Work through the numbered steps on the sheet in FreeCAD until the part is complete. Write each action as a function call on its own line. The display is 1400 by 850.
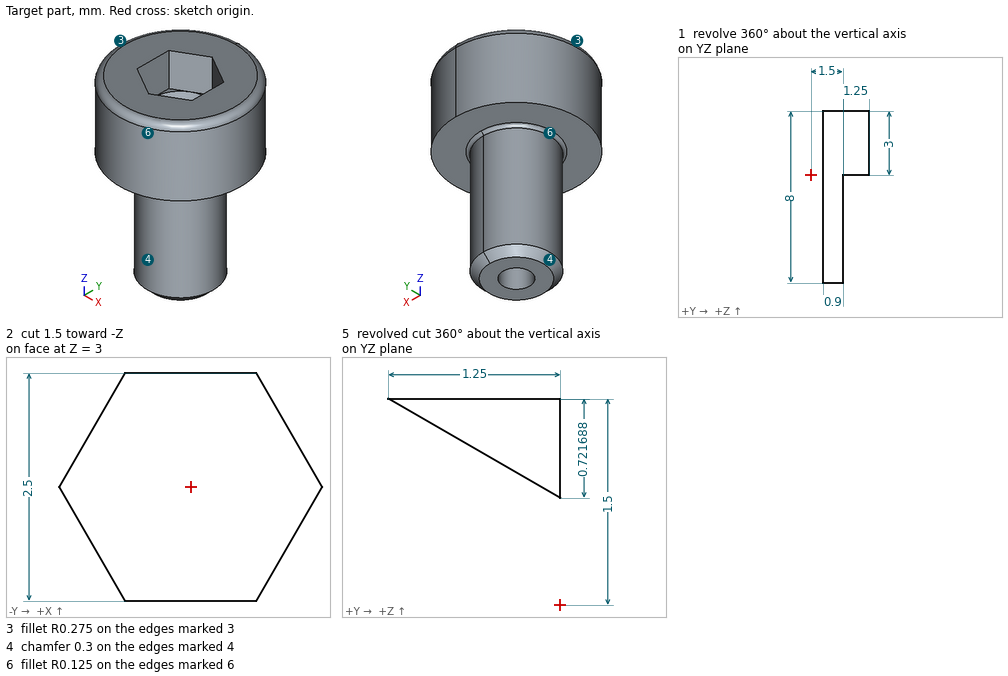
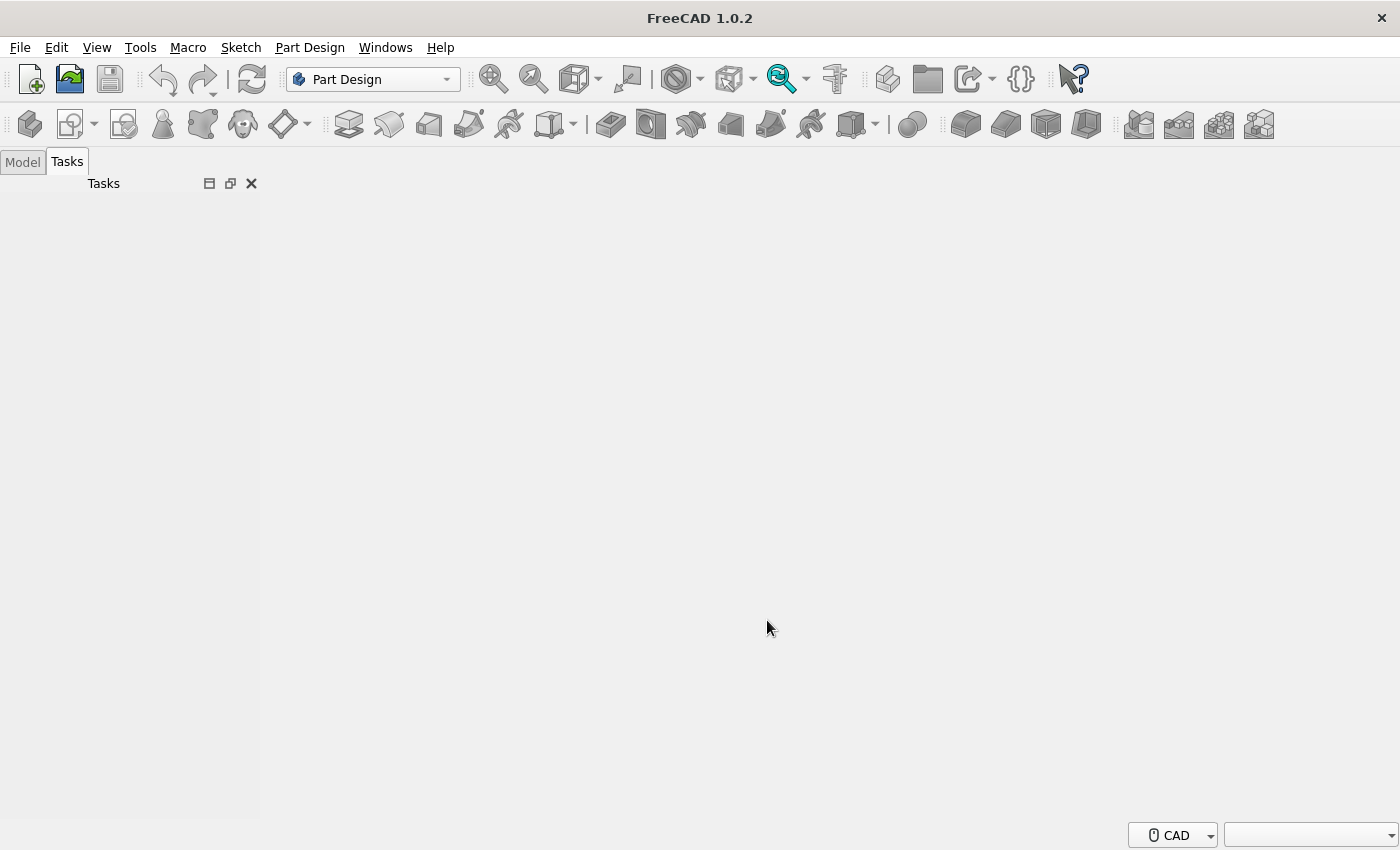
click(30, 80)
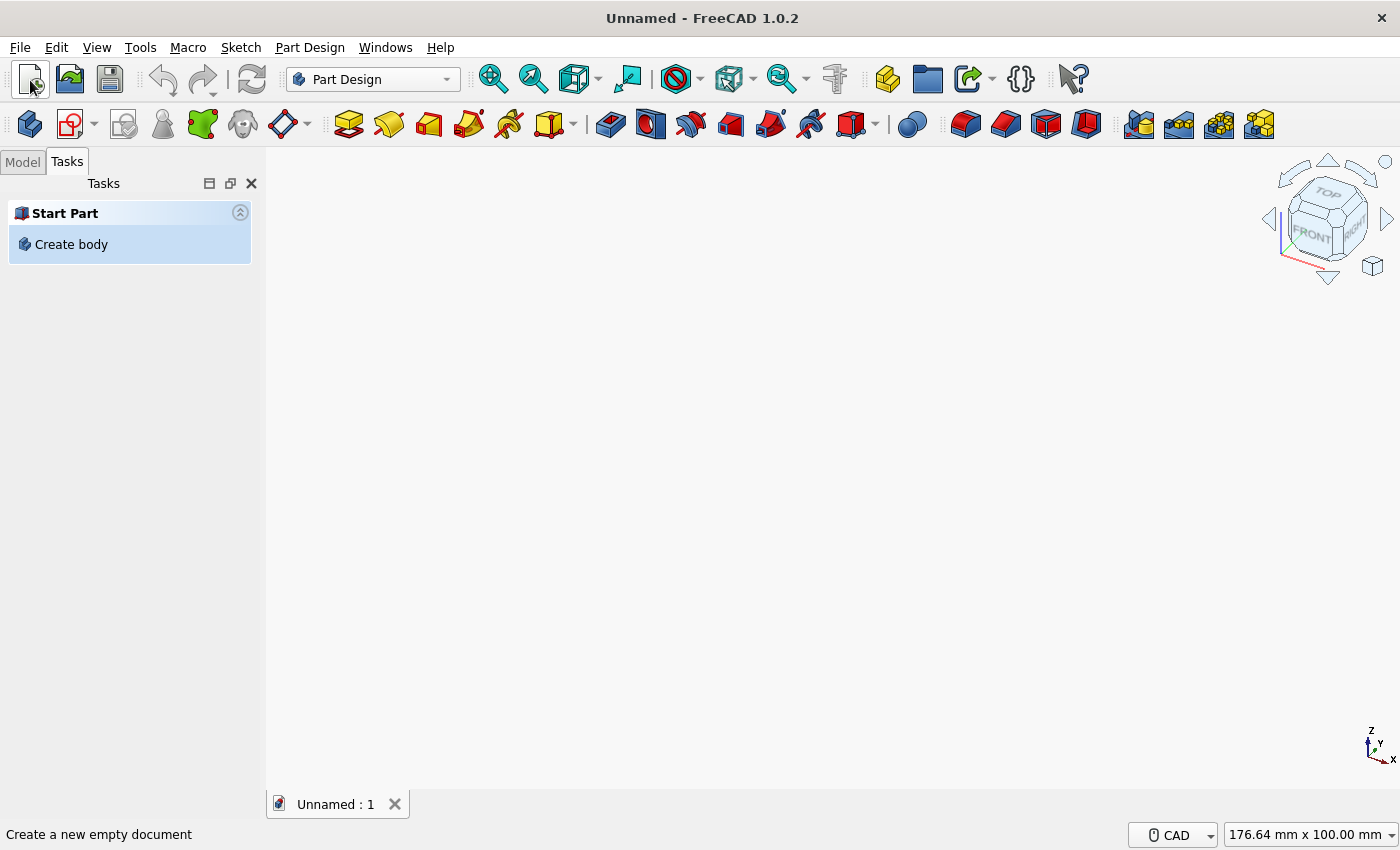
click(70, 124)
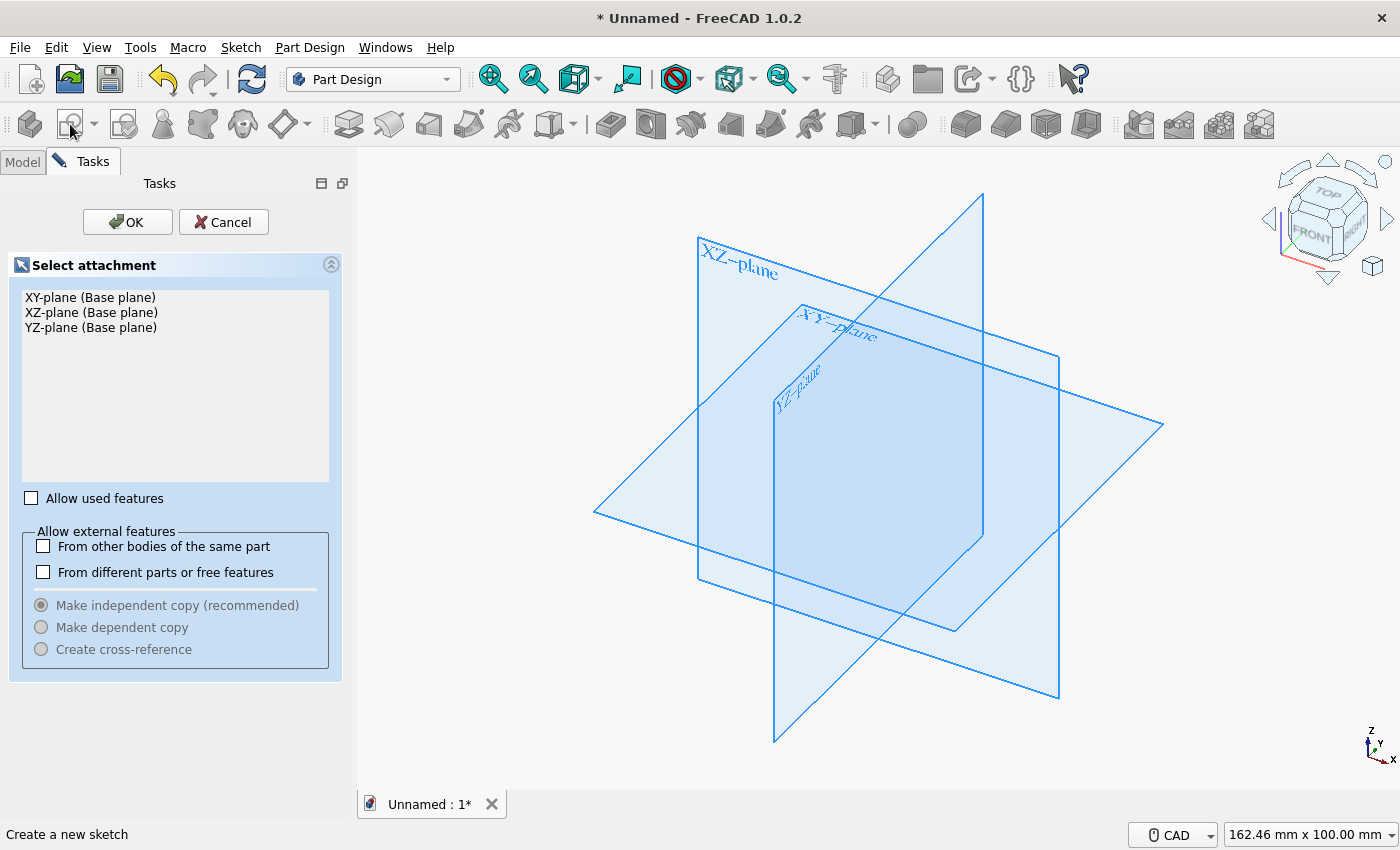
click(82, 328)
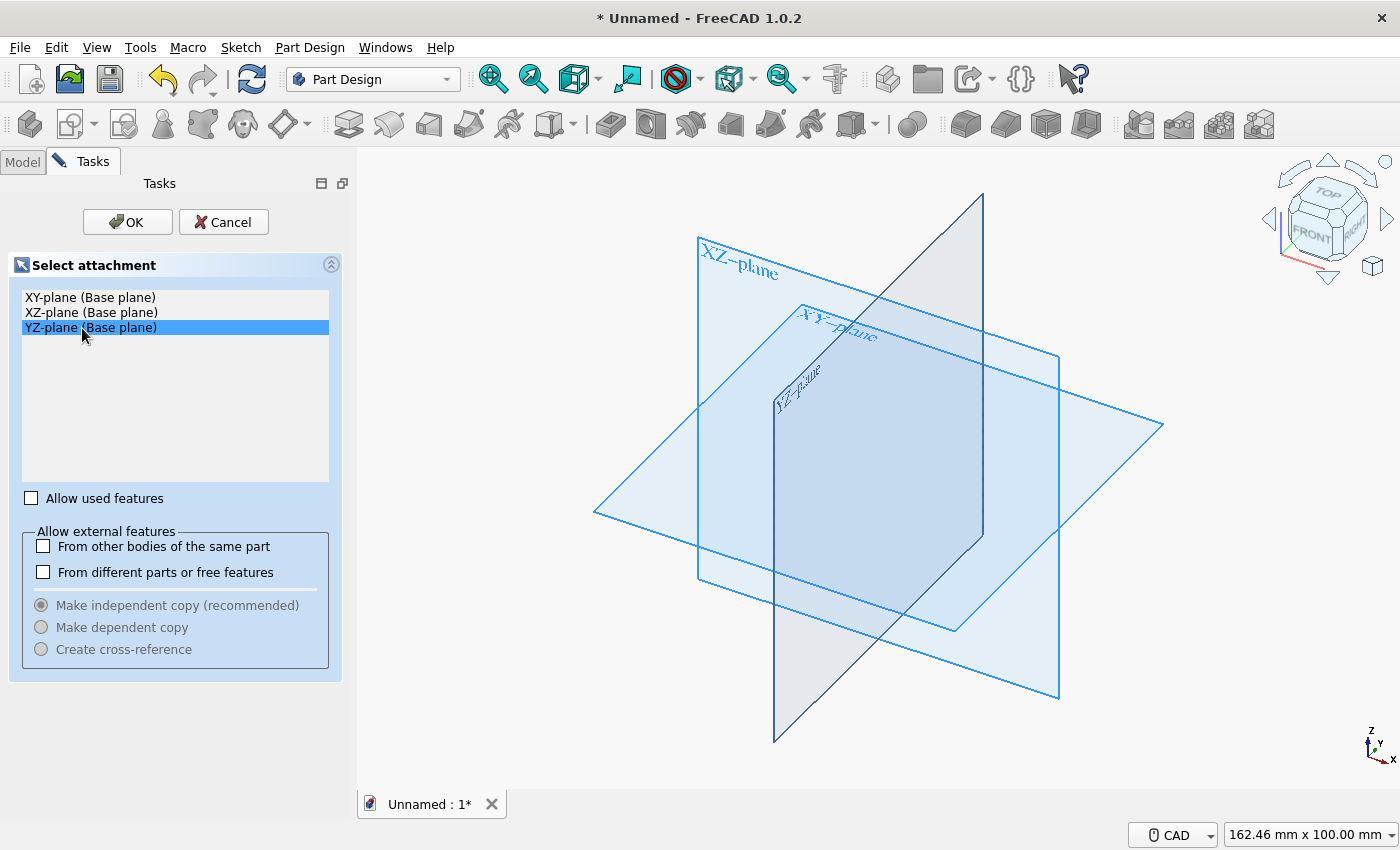
click(128, 222)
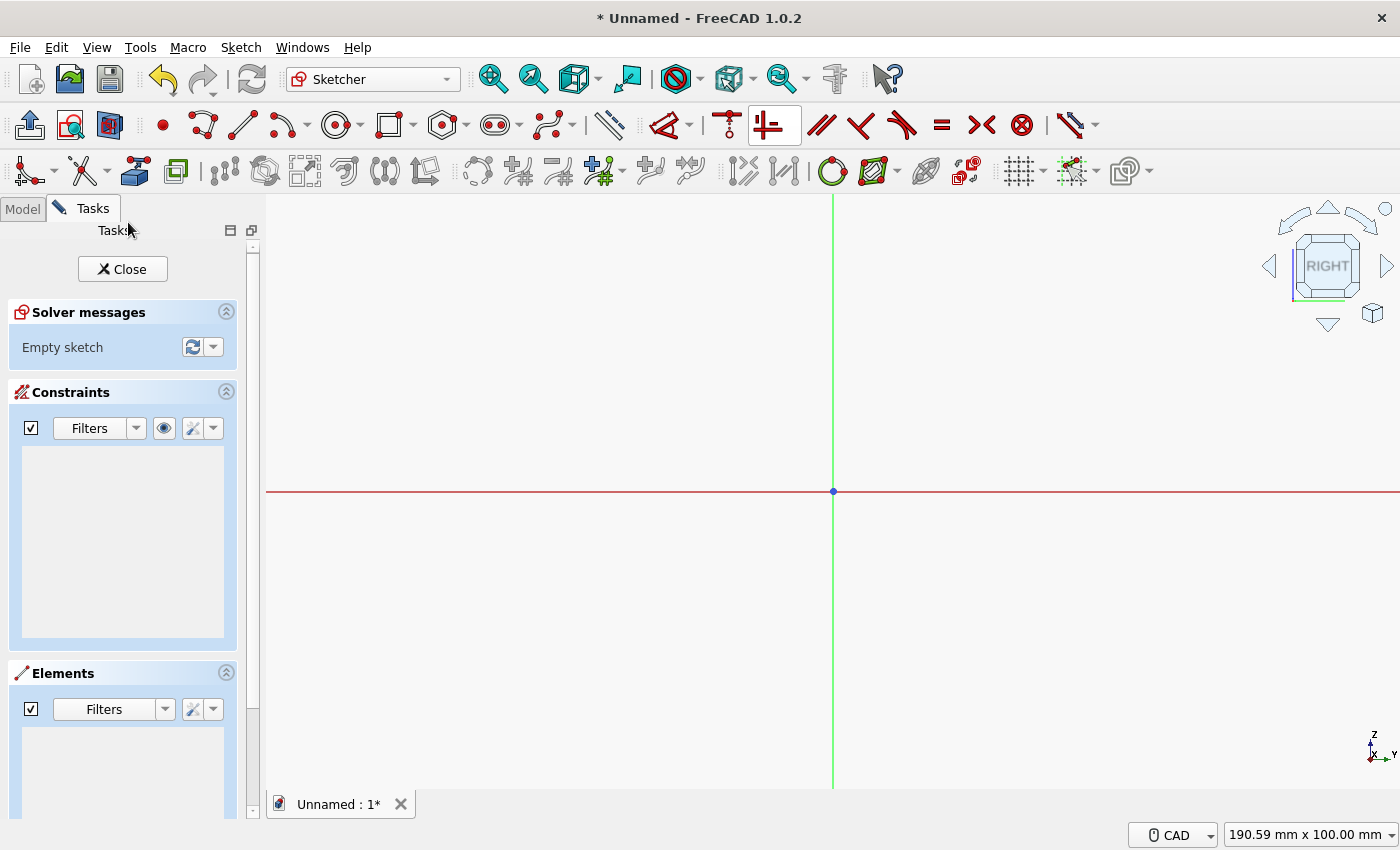
scroll(853, 498, up, 10)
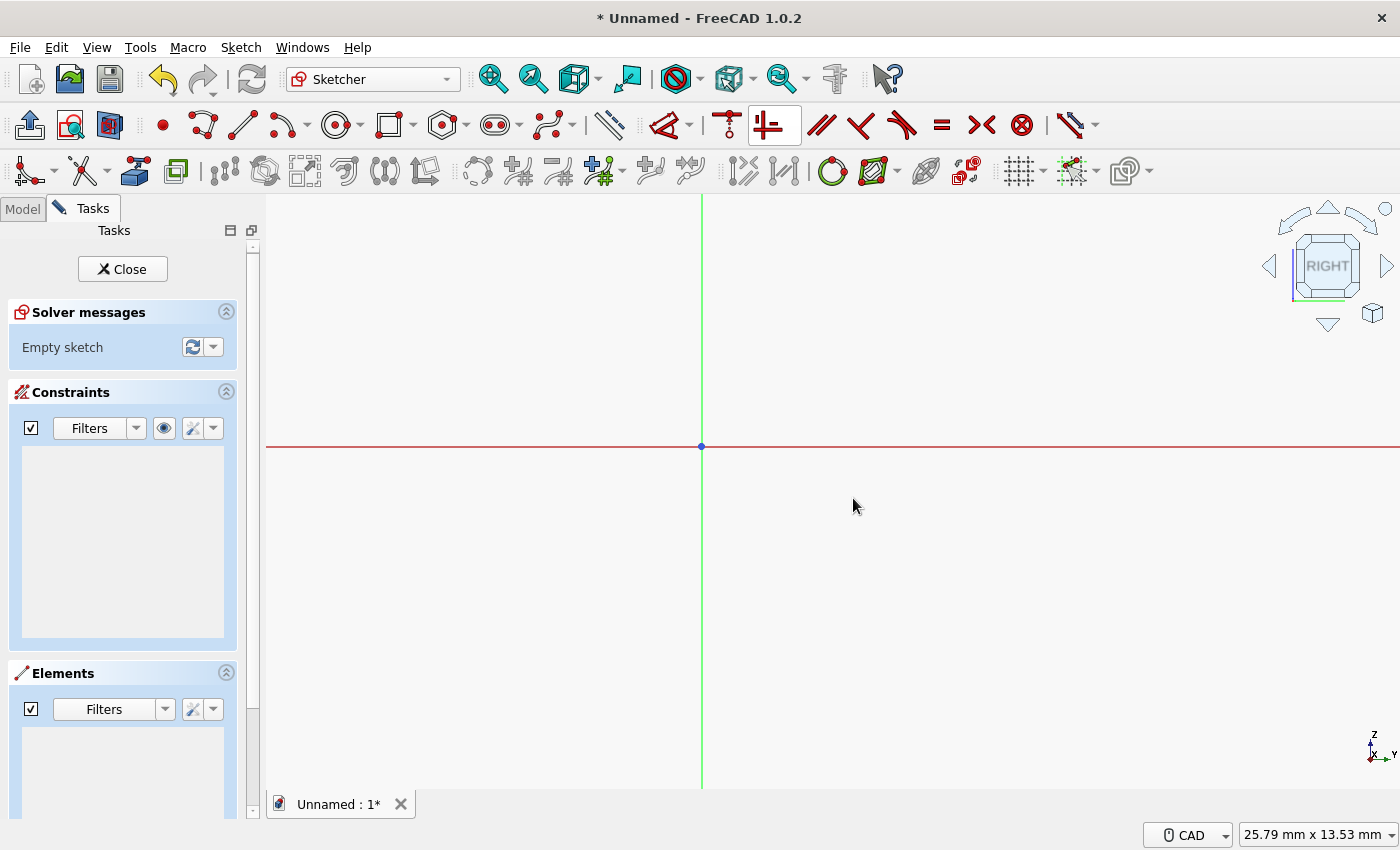
click(204, 126)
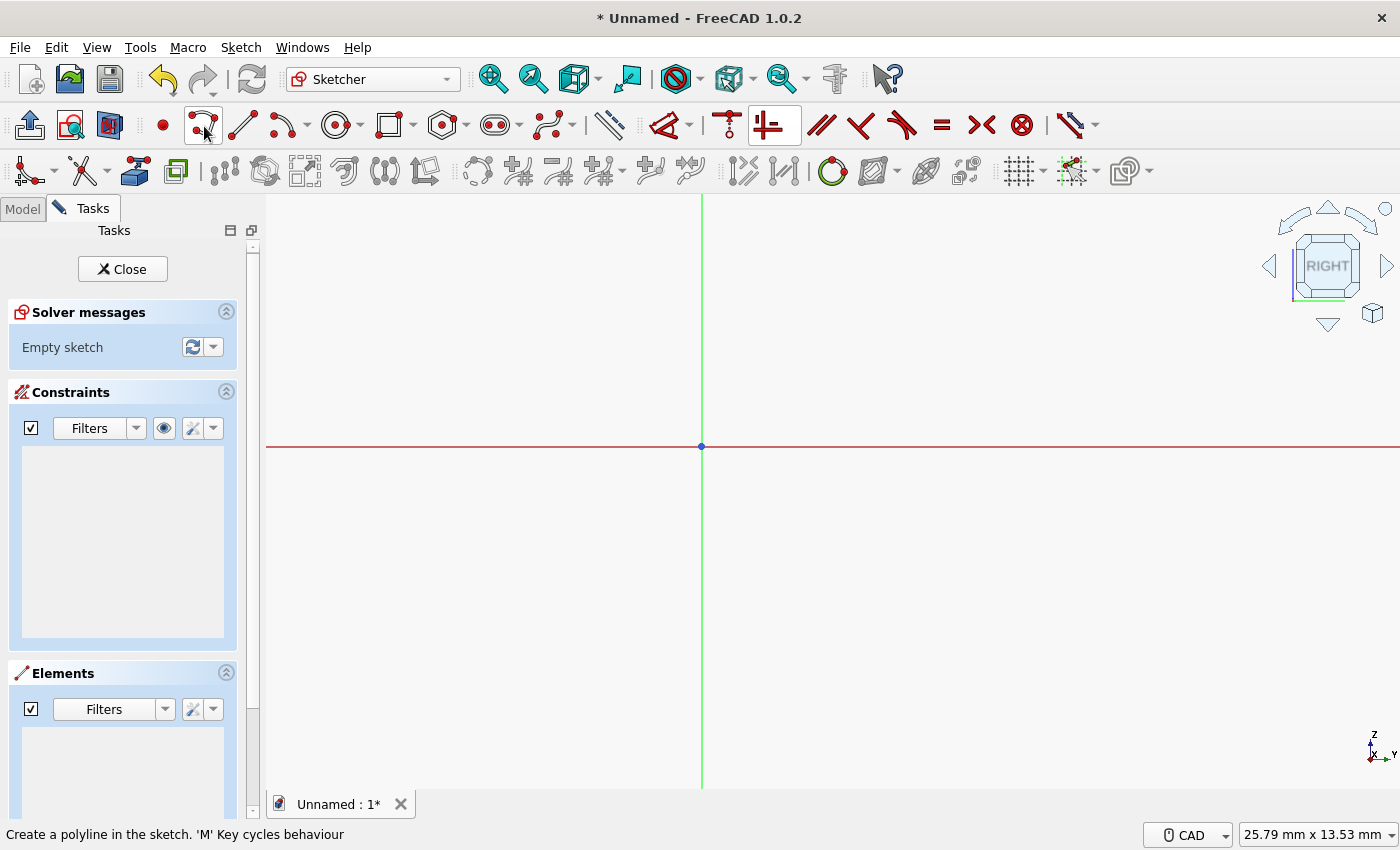
click(768, 447)
click(823, 456)
click(823, 315)
click(728, 315)
click(728, 667)
click(768, 667)
click(768, 447)
key(Escape)
key(Escape)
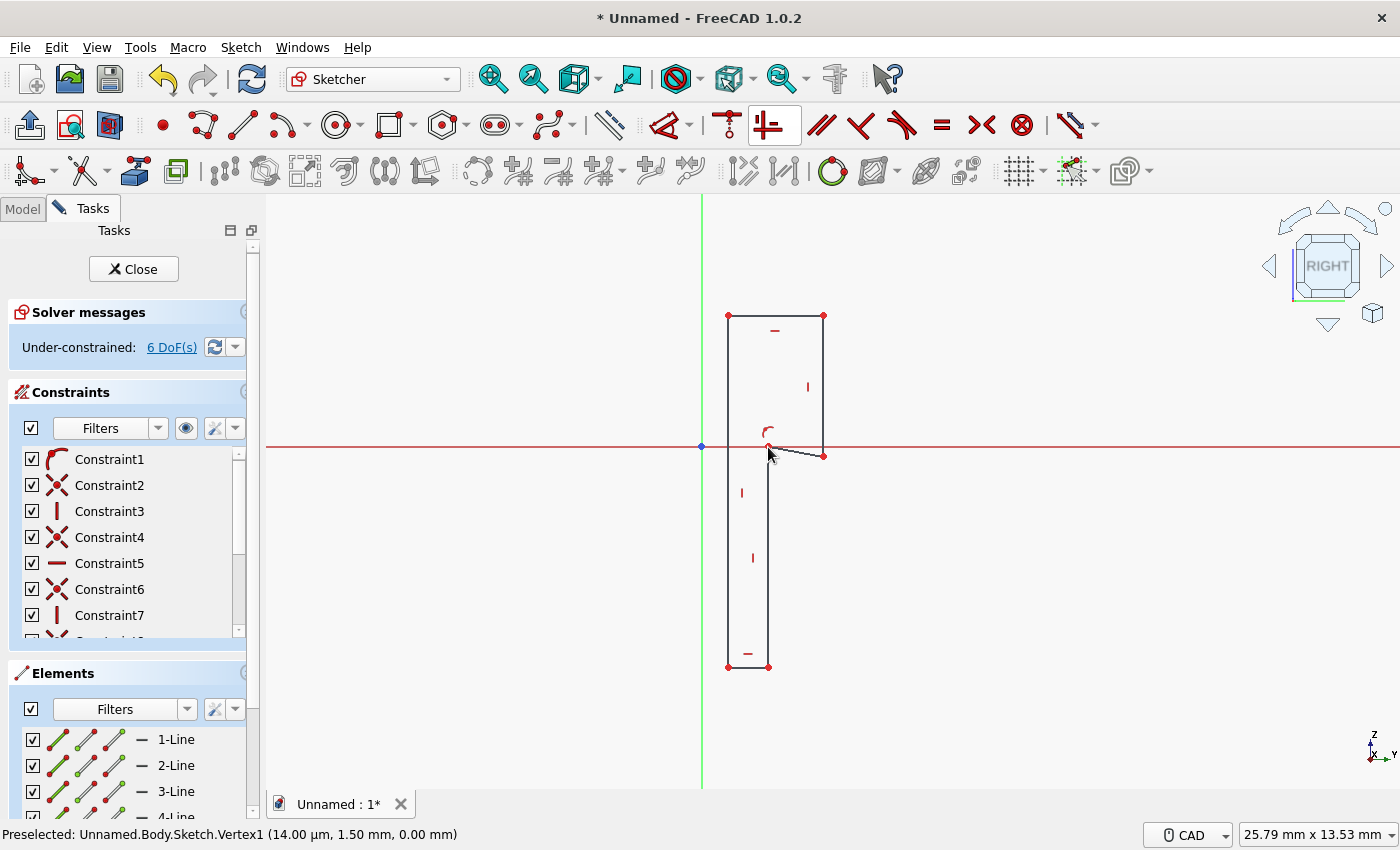
click(785, 450)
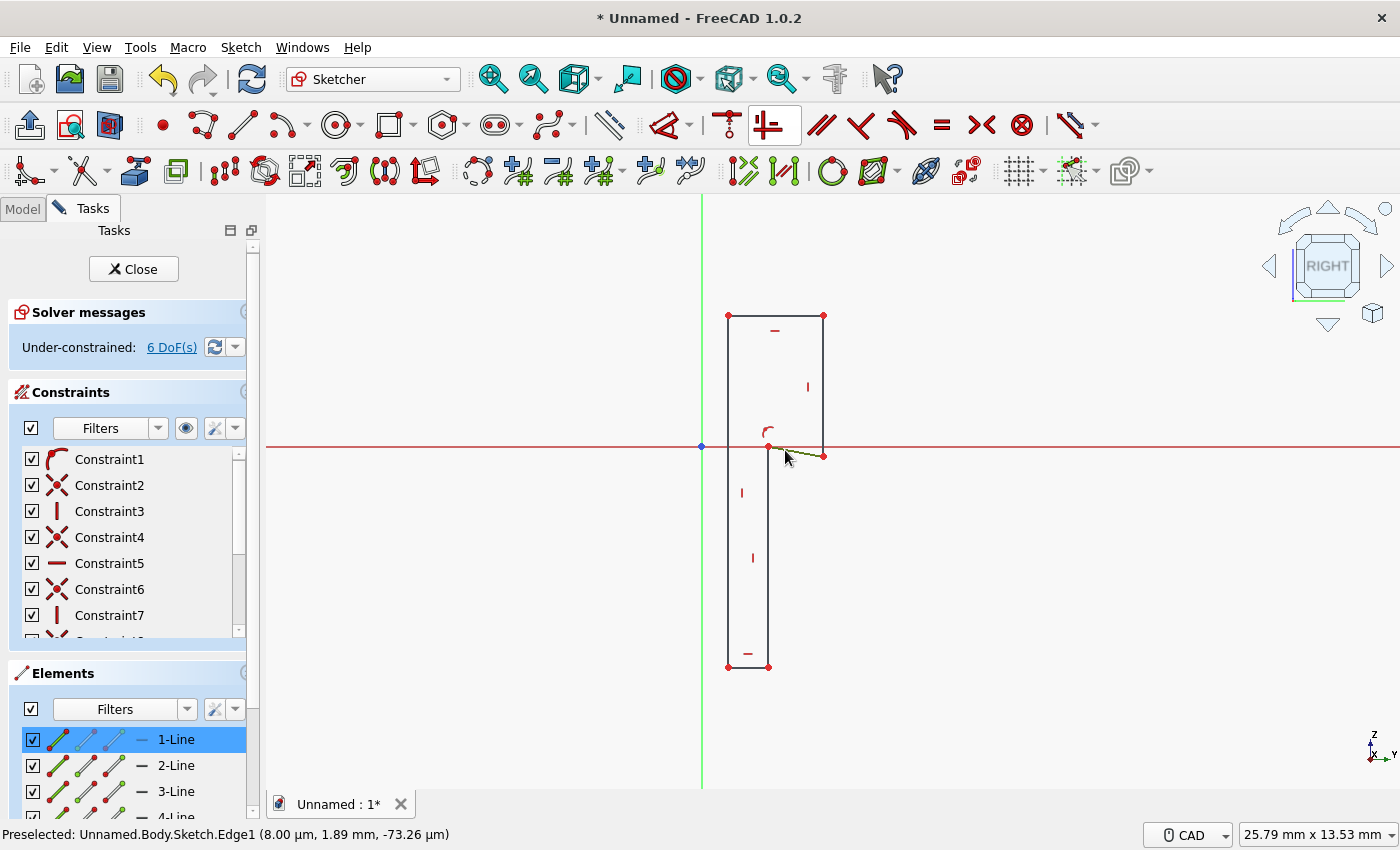
click(796, 126)